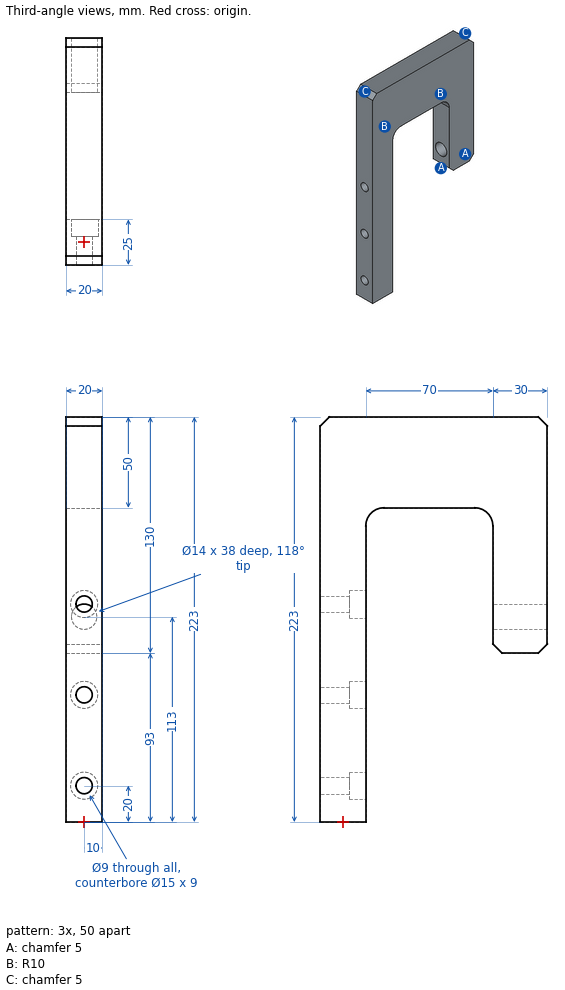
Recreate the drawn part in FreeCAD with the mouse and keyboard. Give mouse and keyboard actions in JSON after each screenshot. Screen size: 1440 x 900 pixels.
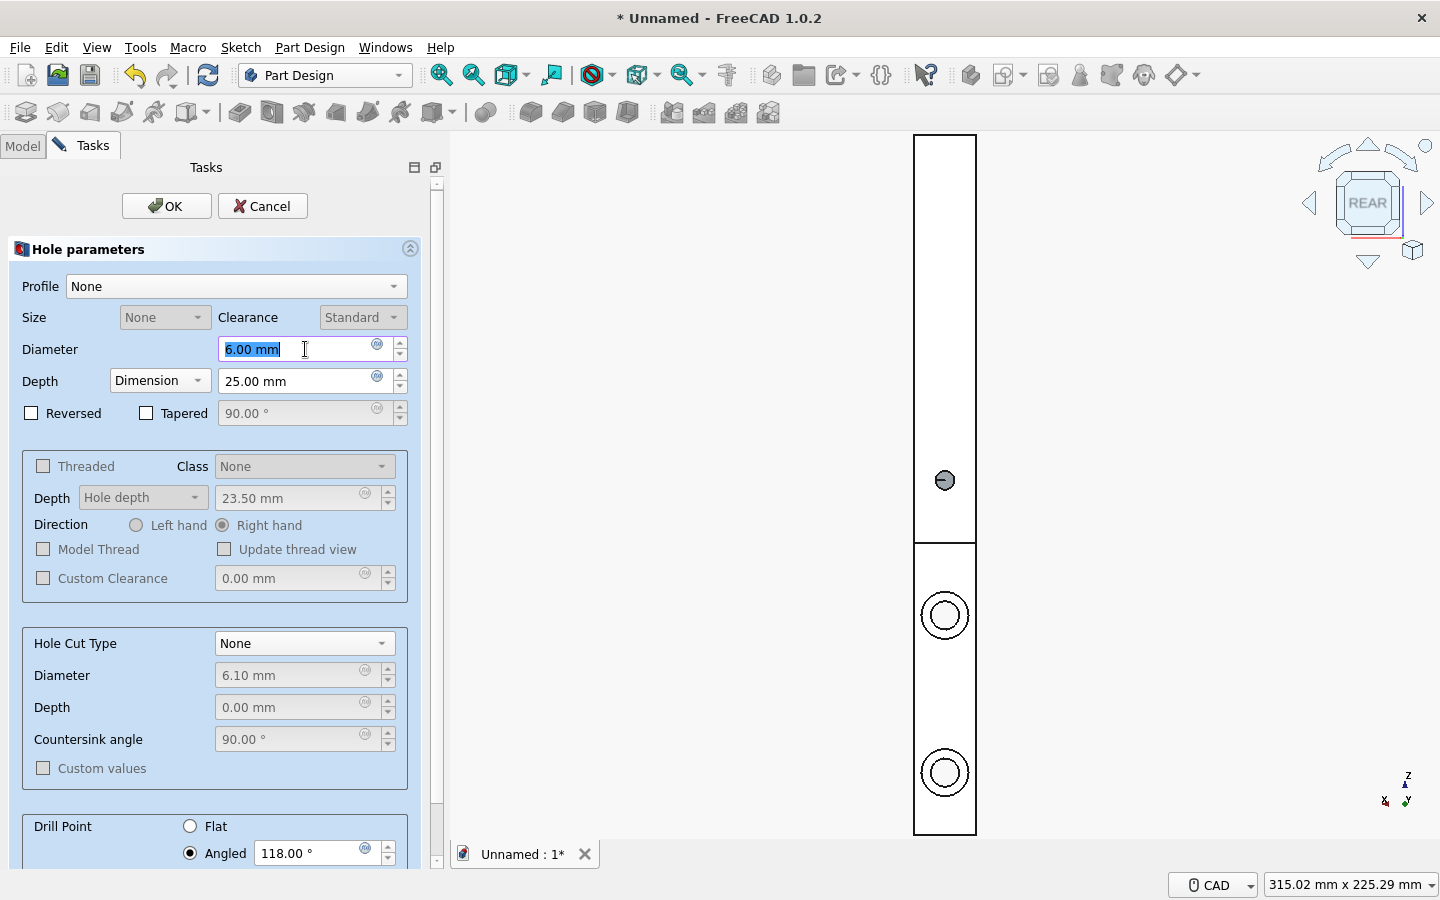
{"action": "type", "text": "14"}
{"action": "key", "text": "Tab"}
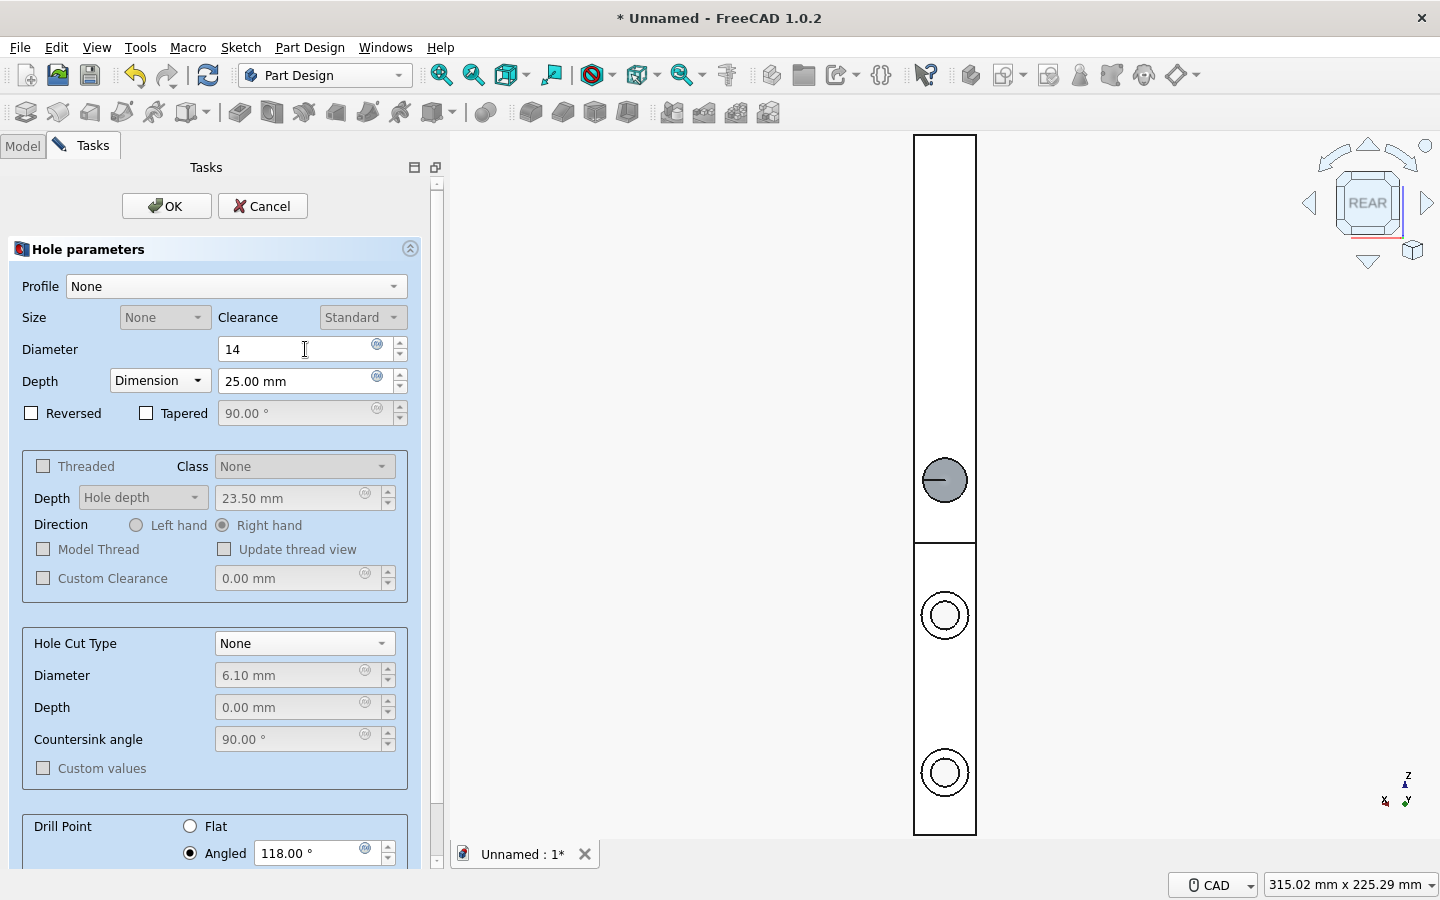
{"action": "triple_click", "coordinate": [305, 381]}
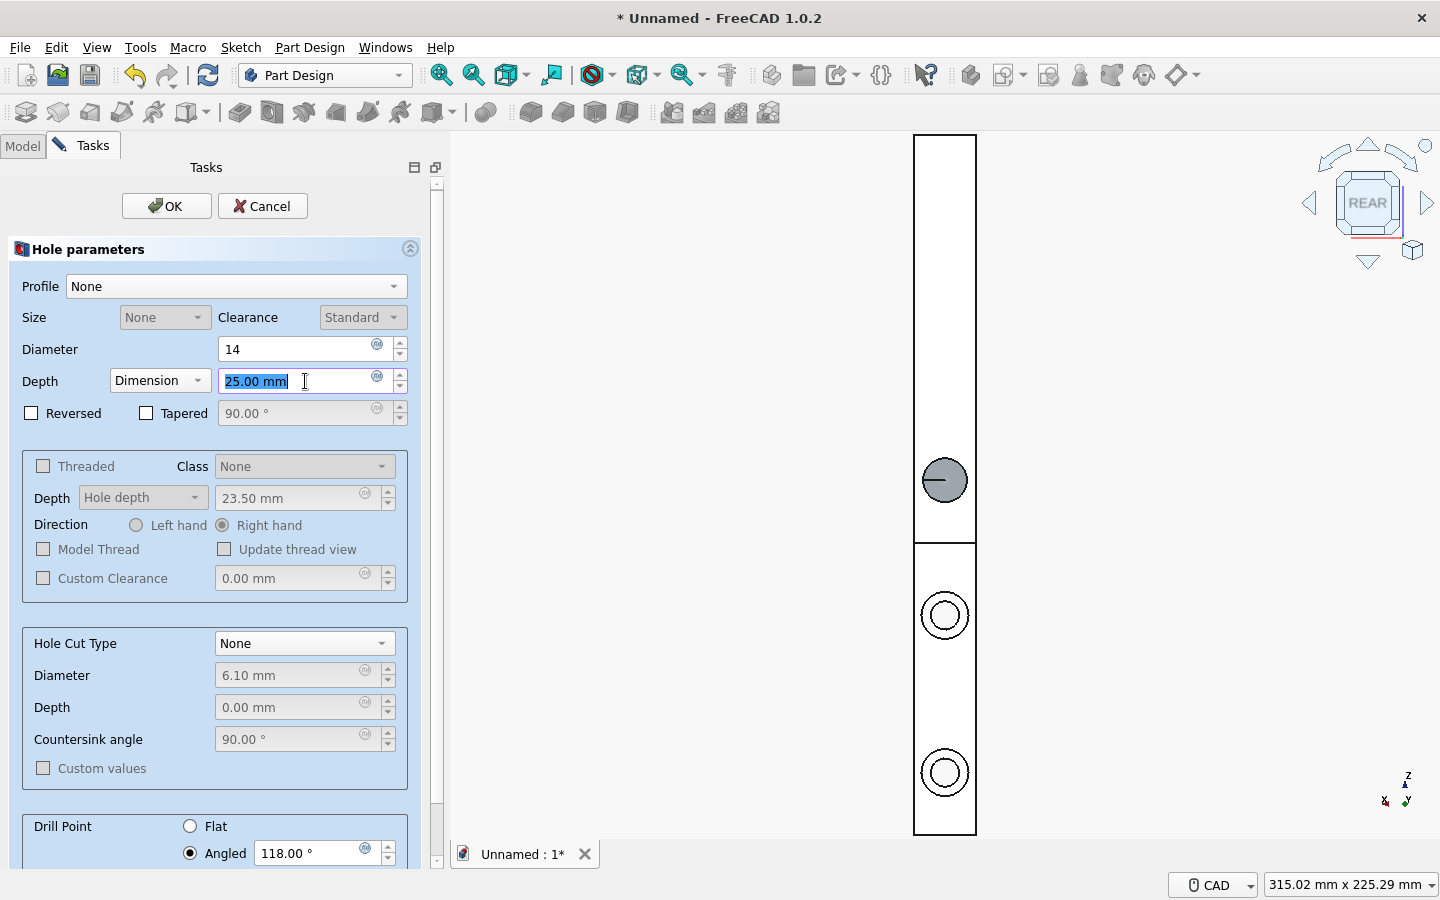
{"action": "type", "text": "38"}
{"action": "key", "text": "Tab"}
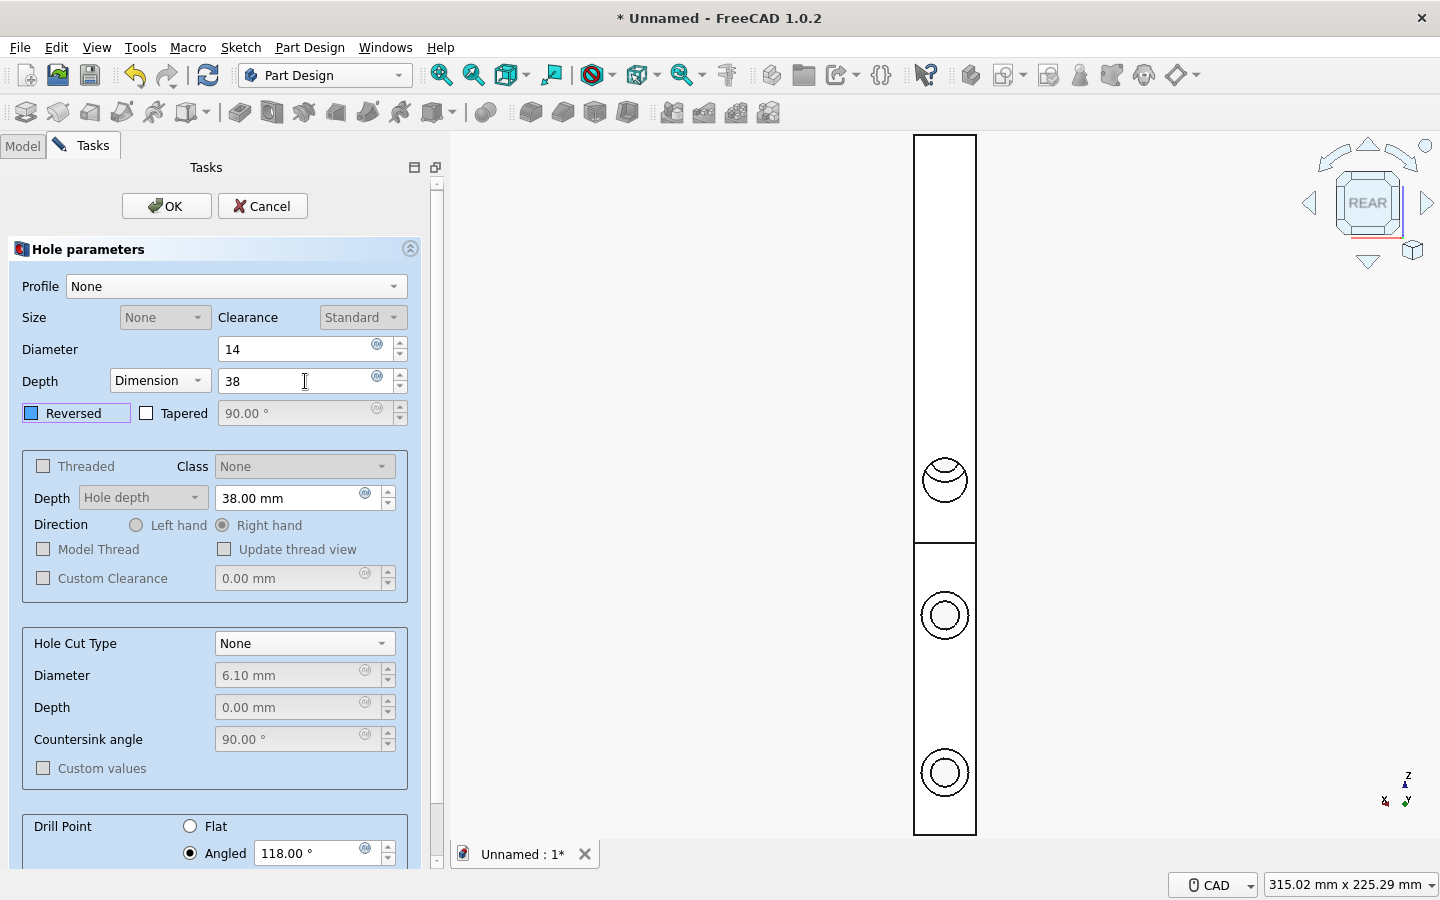
{"action": "left_click", "coordinate": [167, 206]}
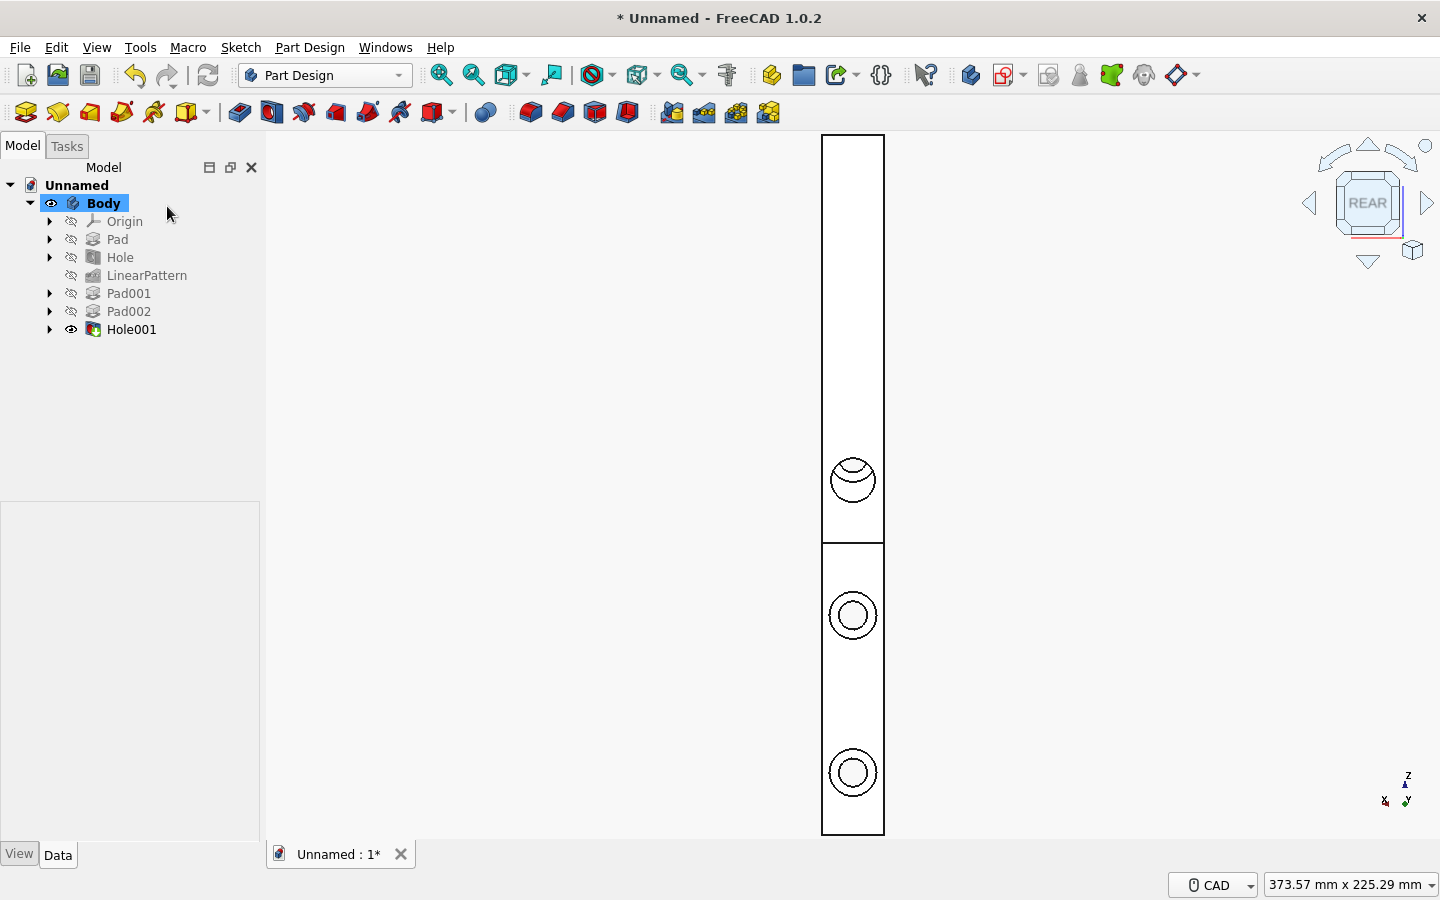
{"action": "left_click", "coordinate": [853, 542]}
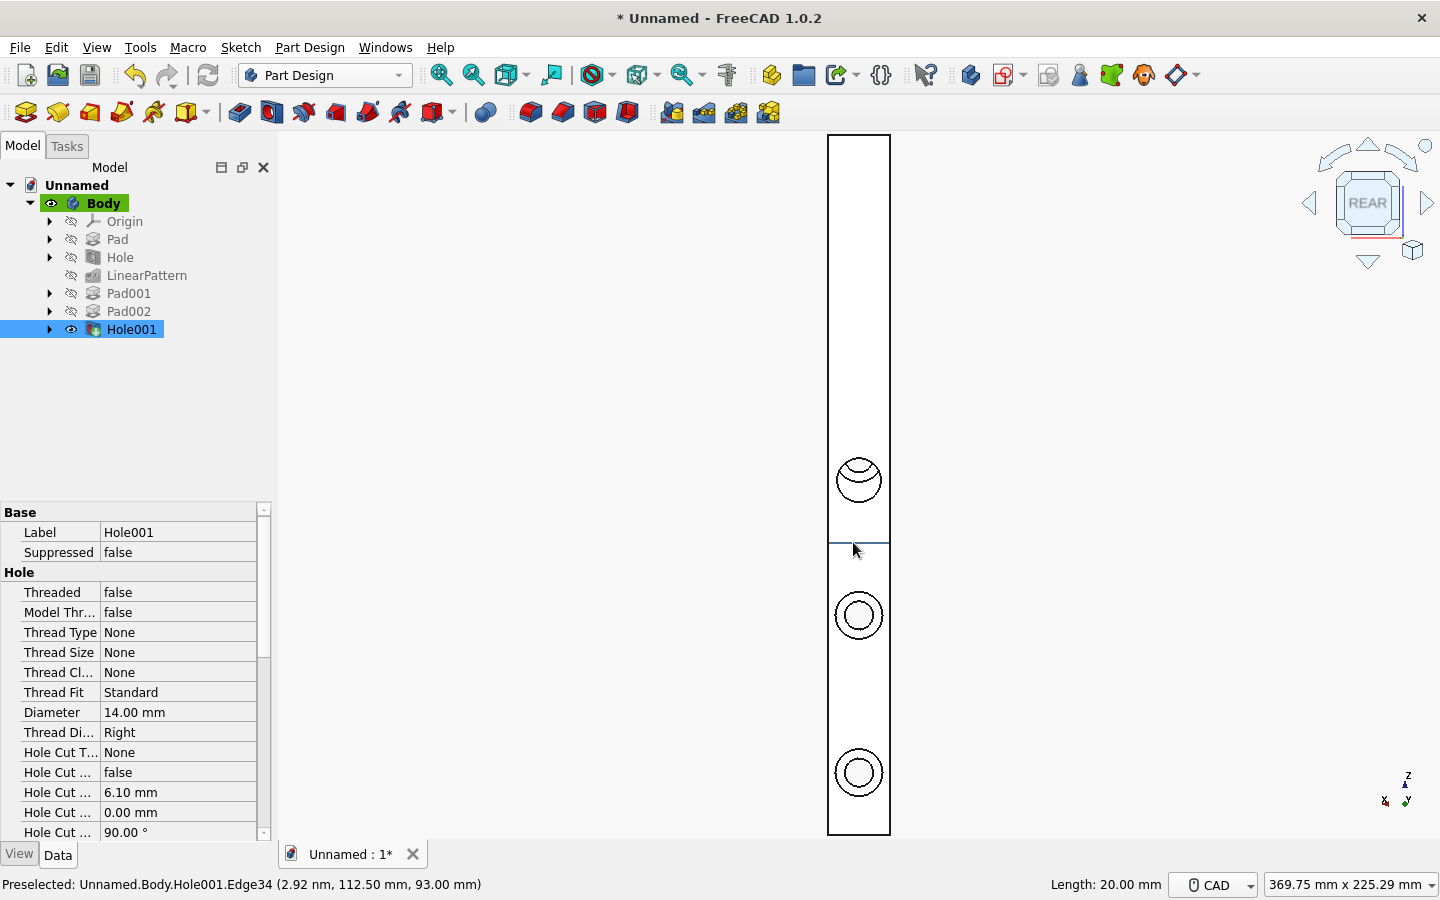
{"action": "key", "text": "0"}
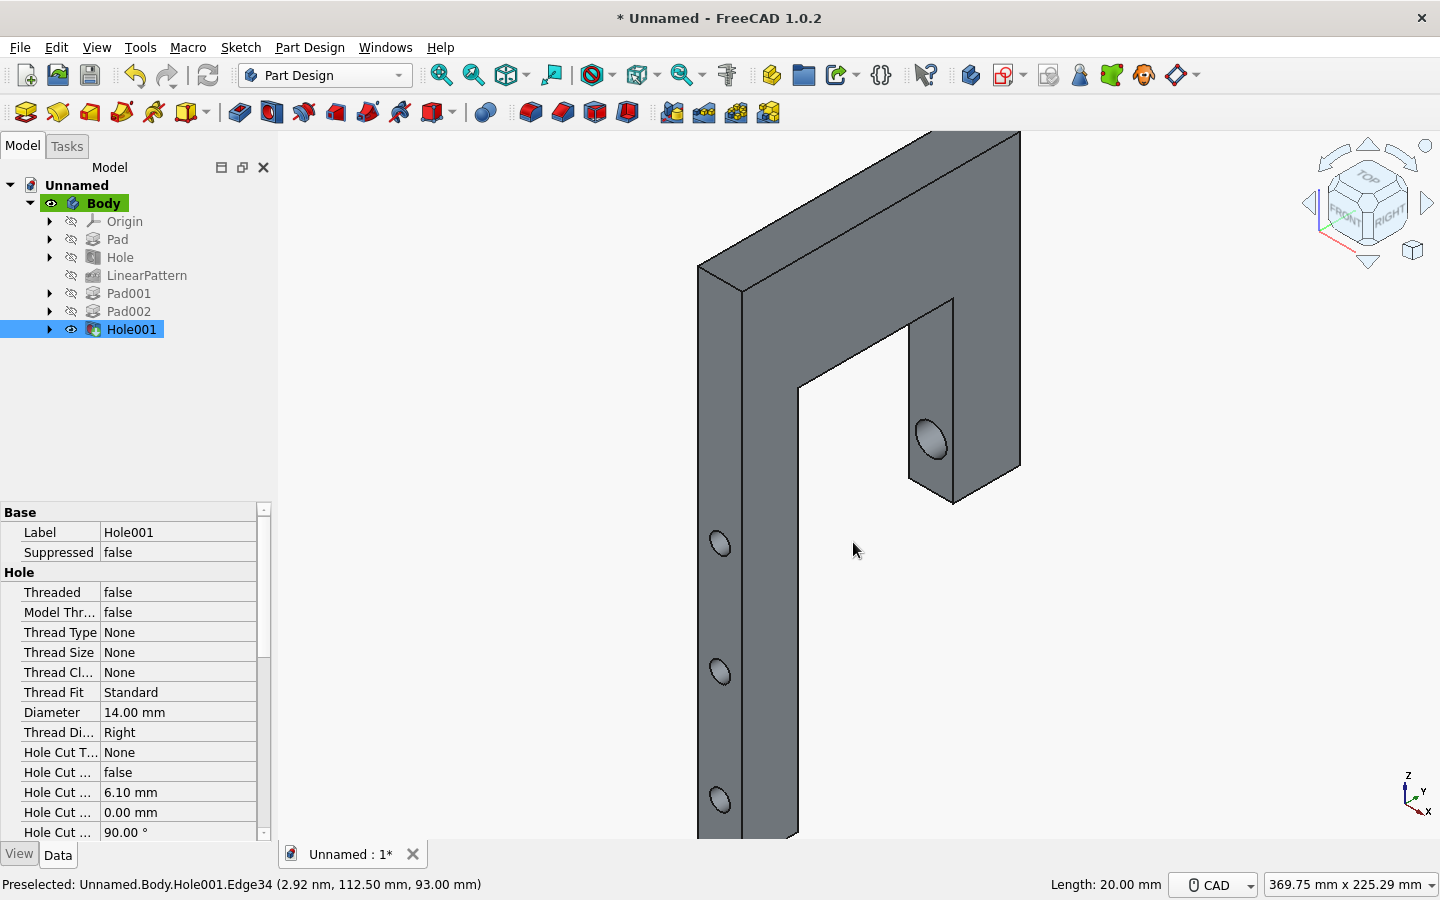
{"action": "left_click", "coordinate": [442, 76]}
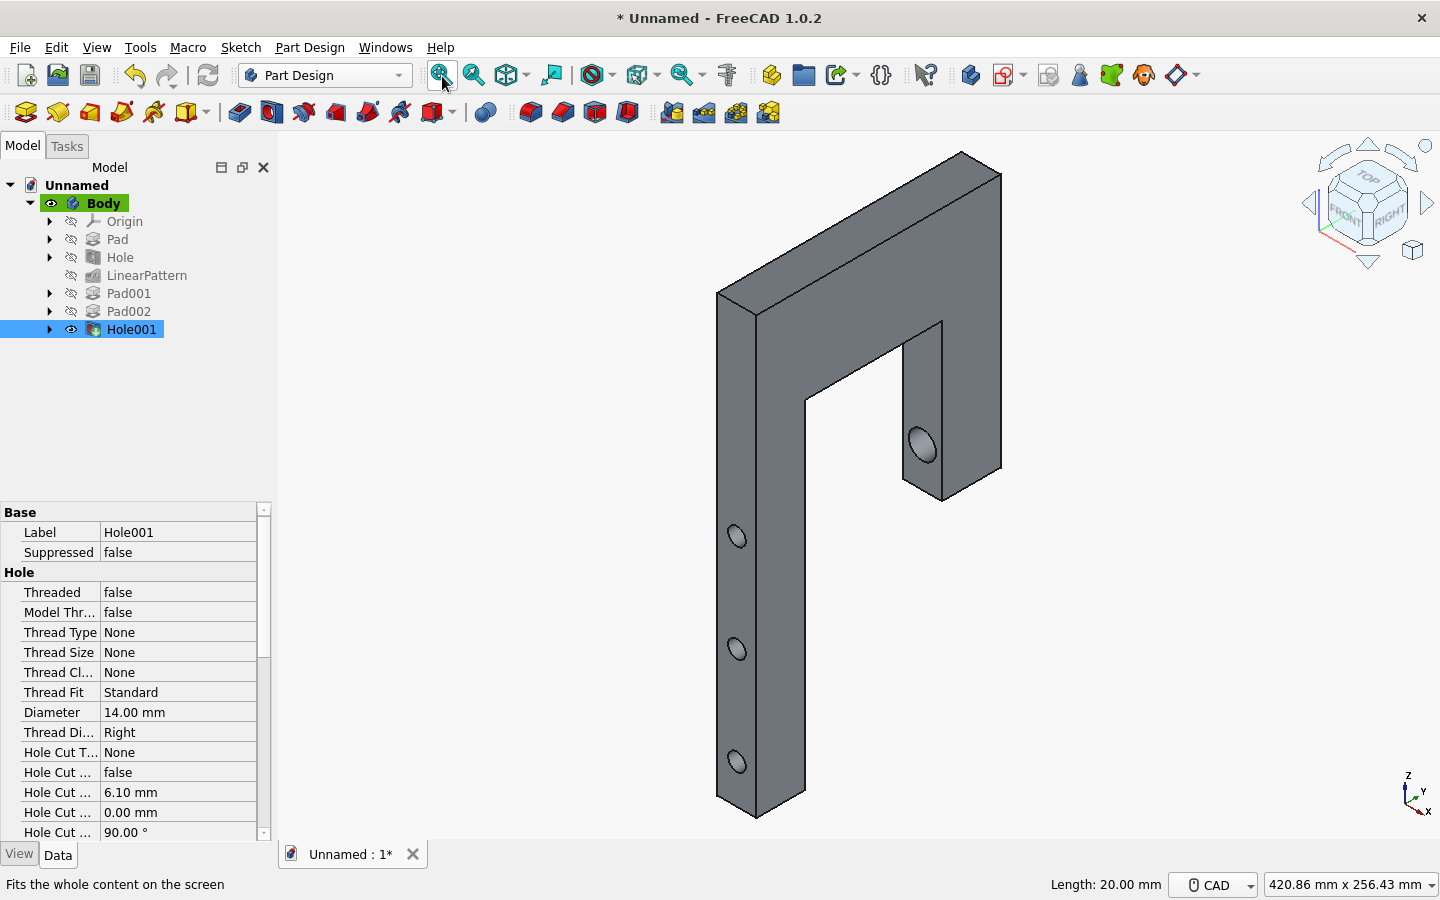
{"action": "key", "text": "2"}